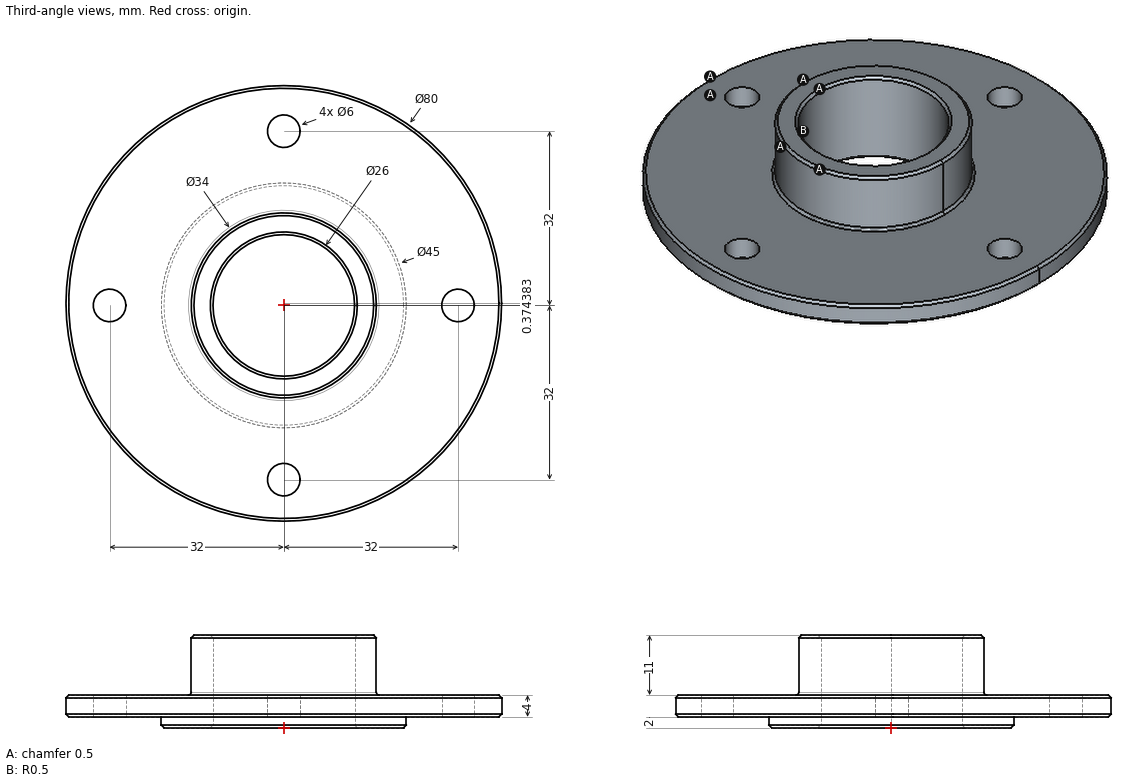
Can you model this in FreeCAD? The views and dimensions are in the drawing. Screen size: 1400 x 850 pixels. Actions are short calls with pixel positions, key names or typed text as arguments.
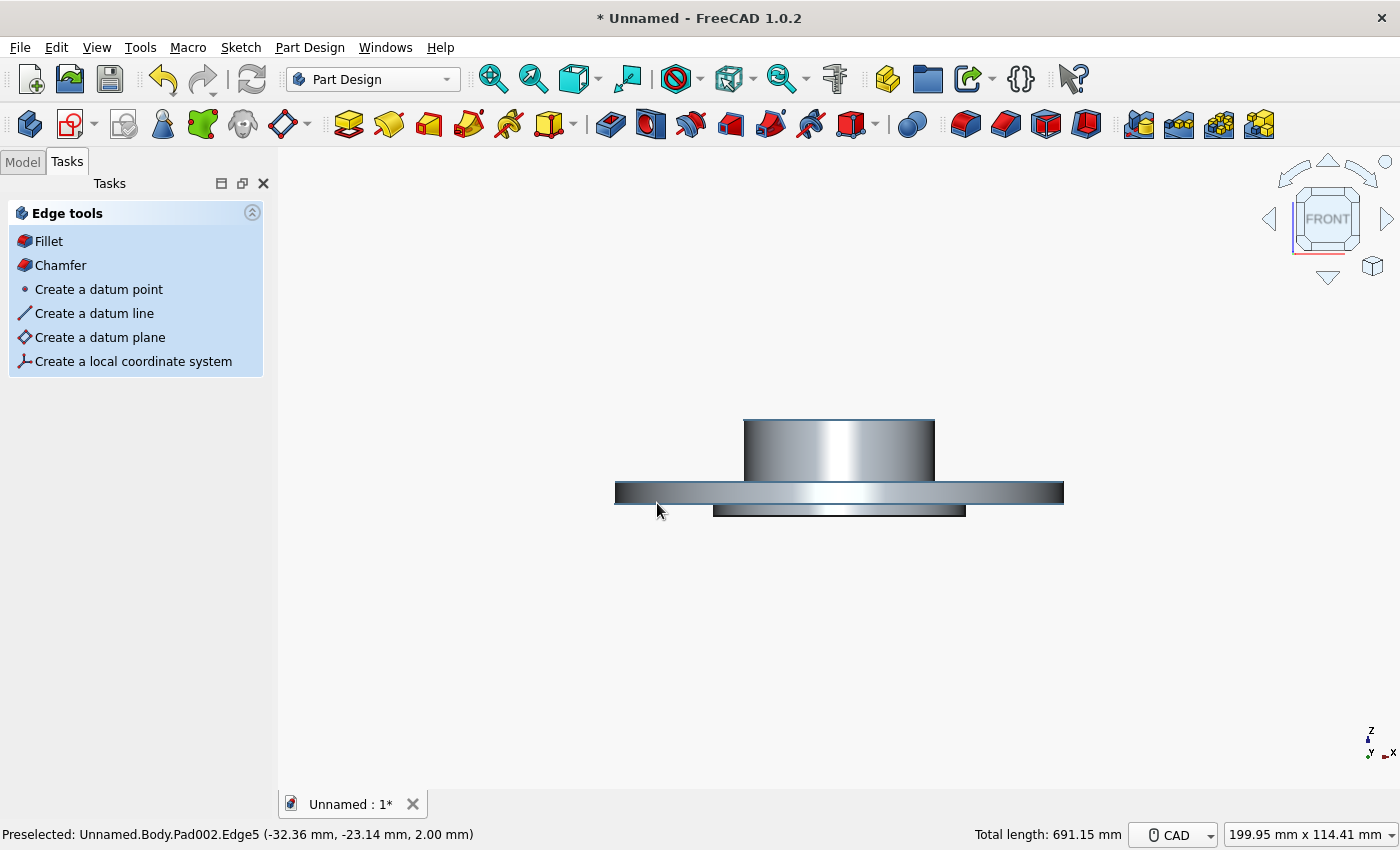
click(737, 515, ctrl)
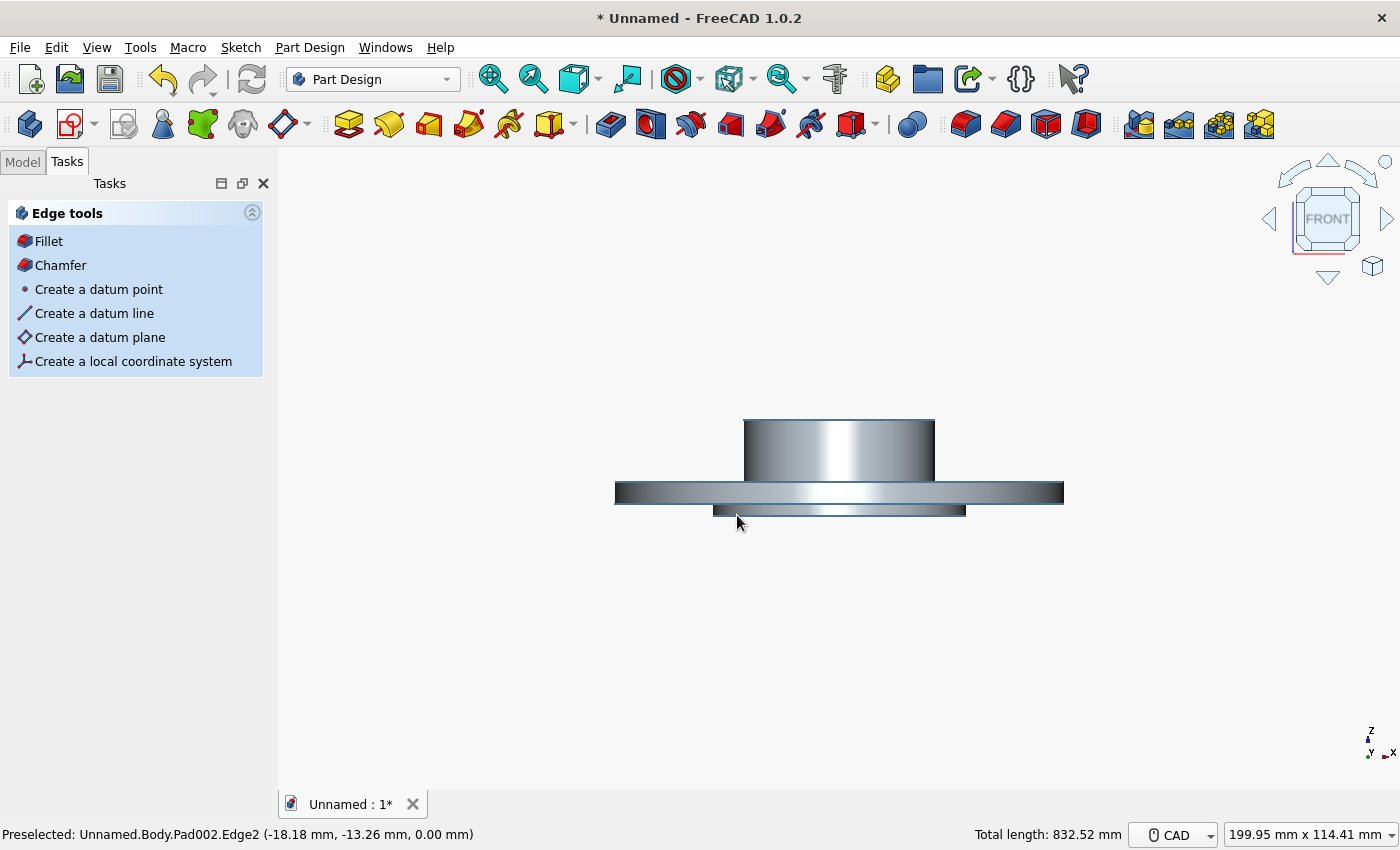
key(3)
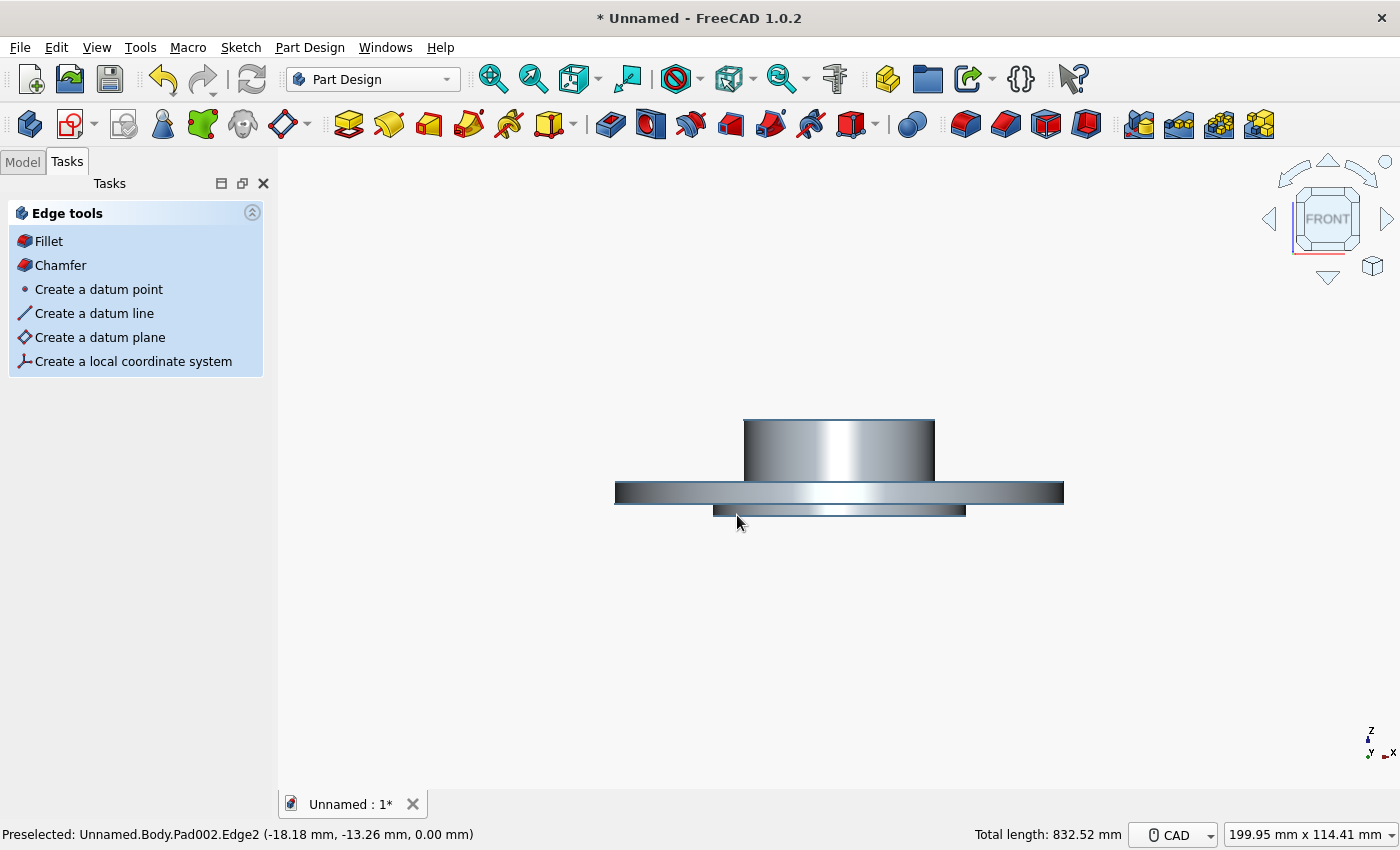
click(494, 80)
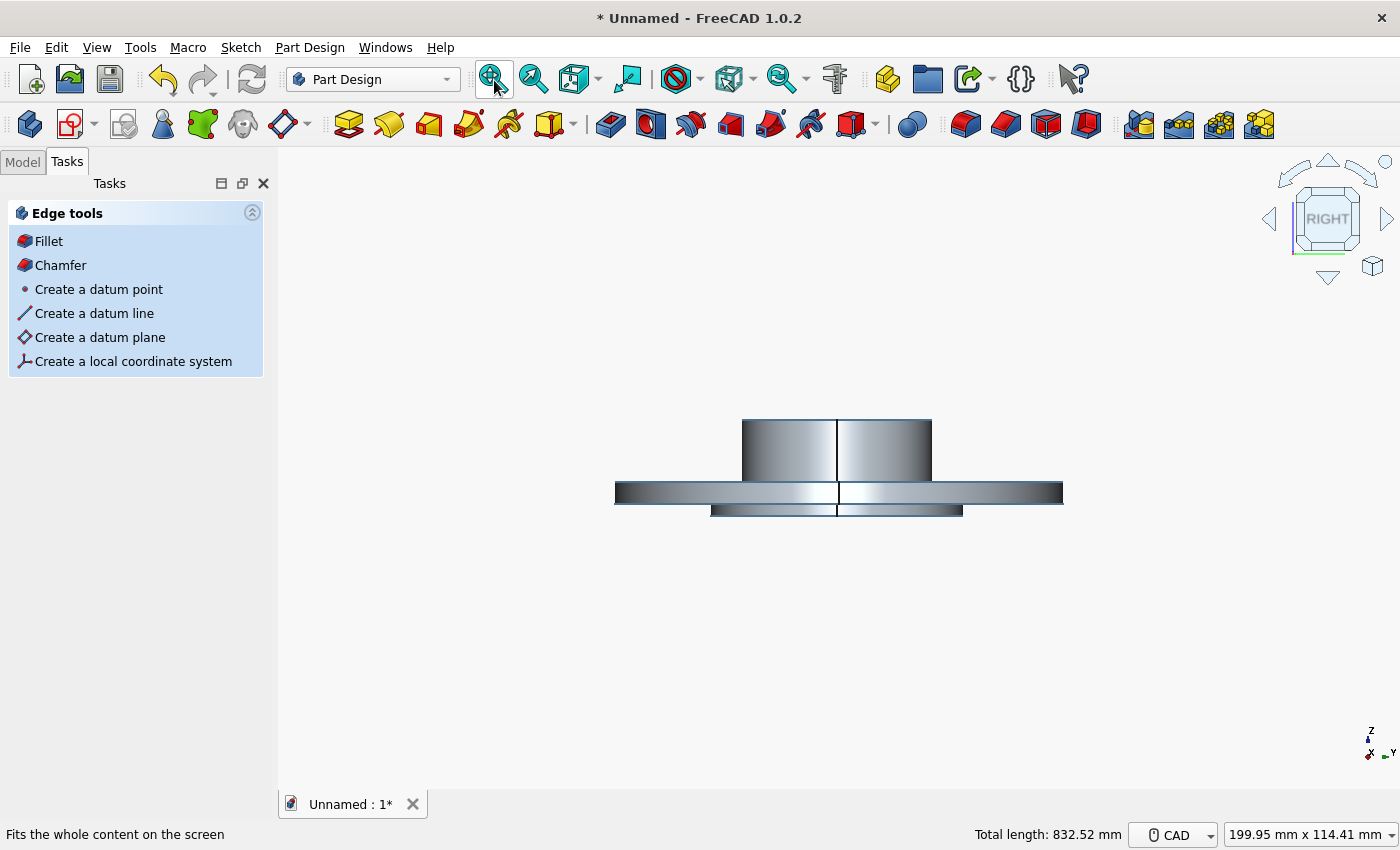
key(5)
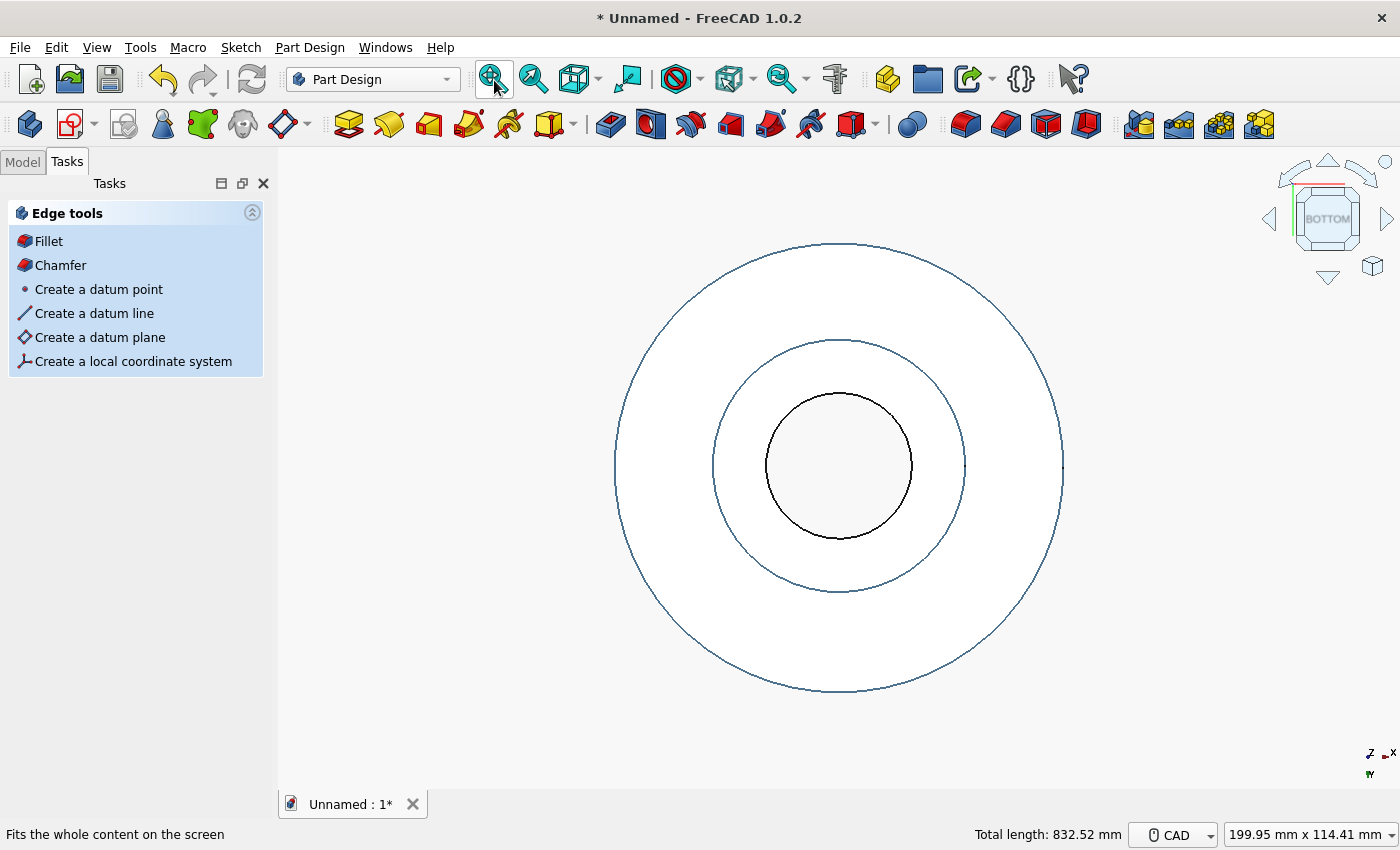
click(766, 465, ctrl)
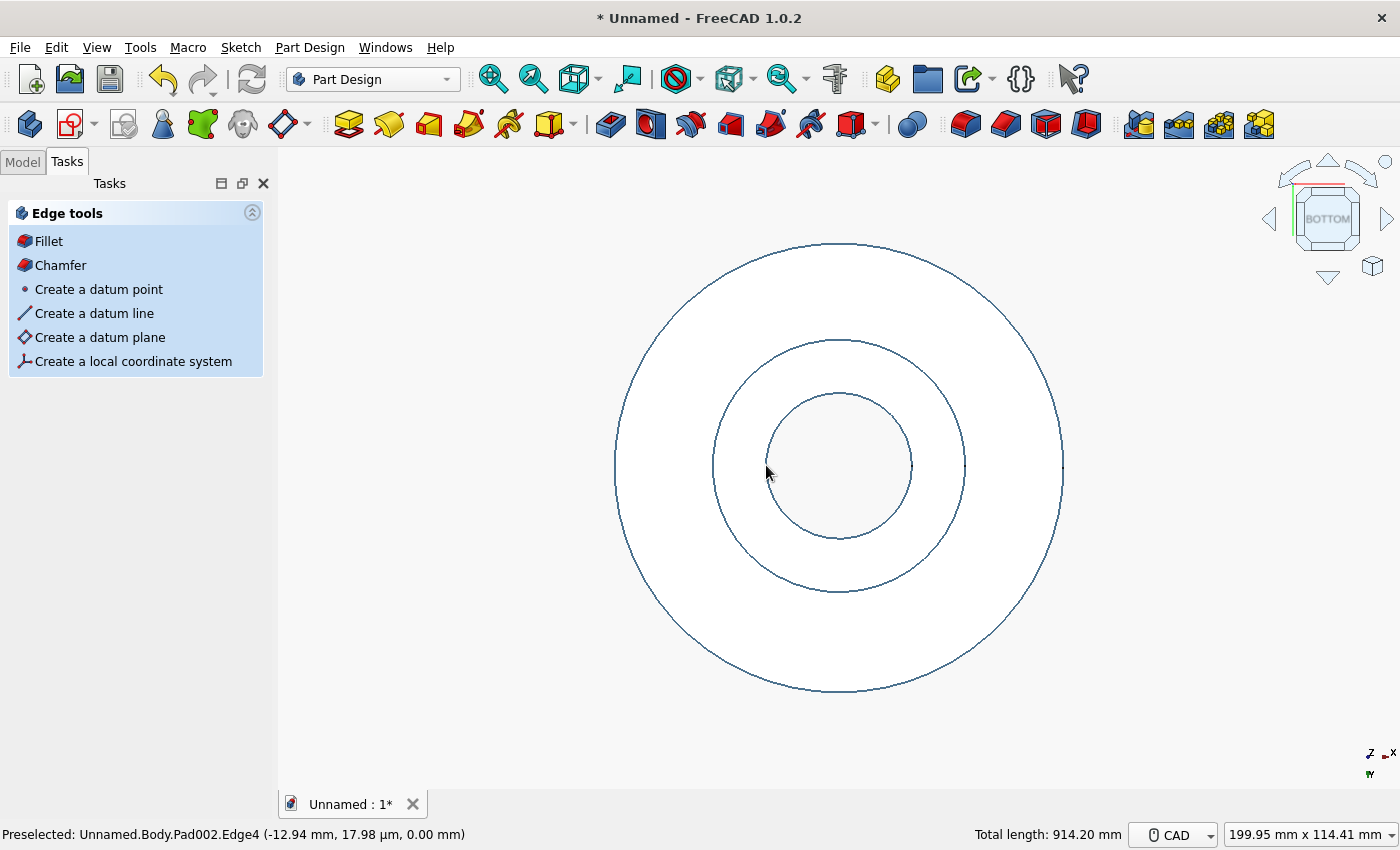
click(1006, 124)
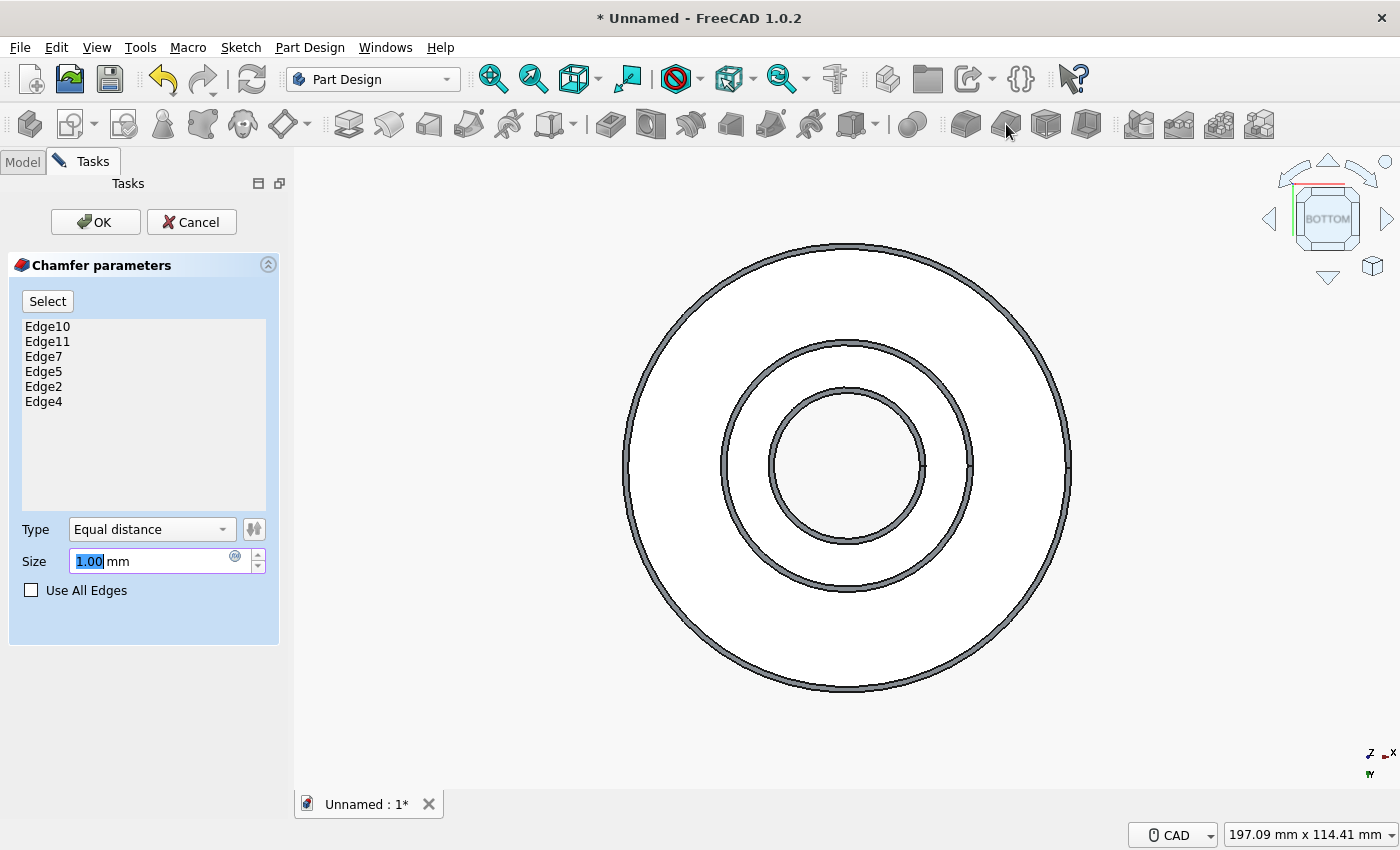
text(0.5)
key(Tab)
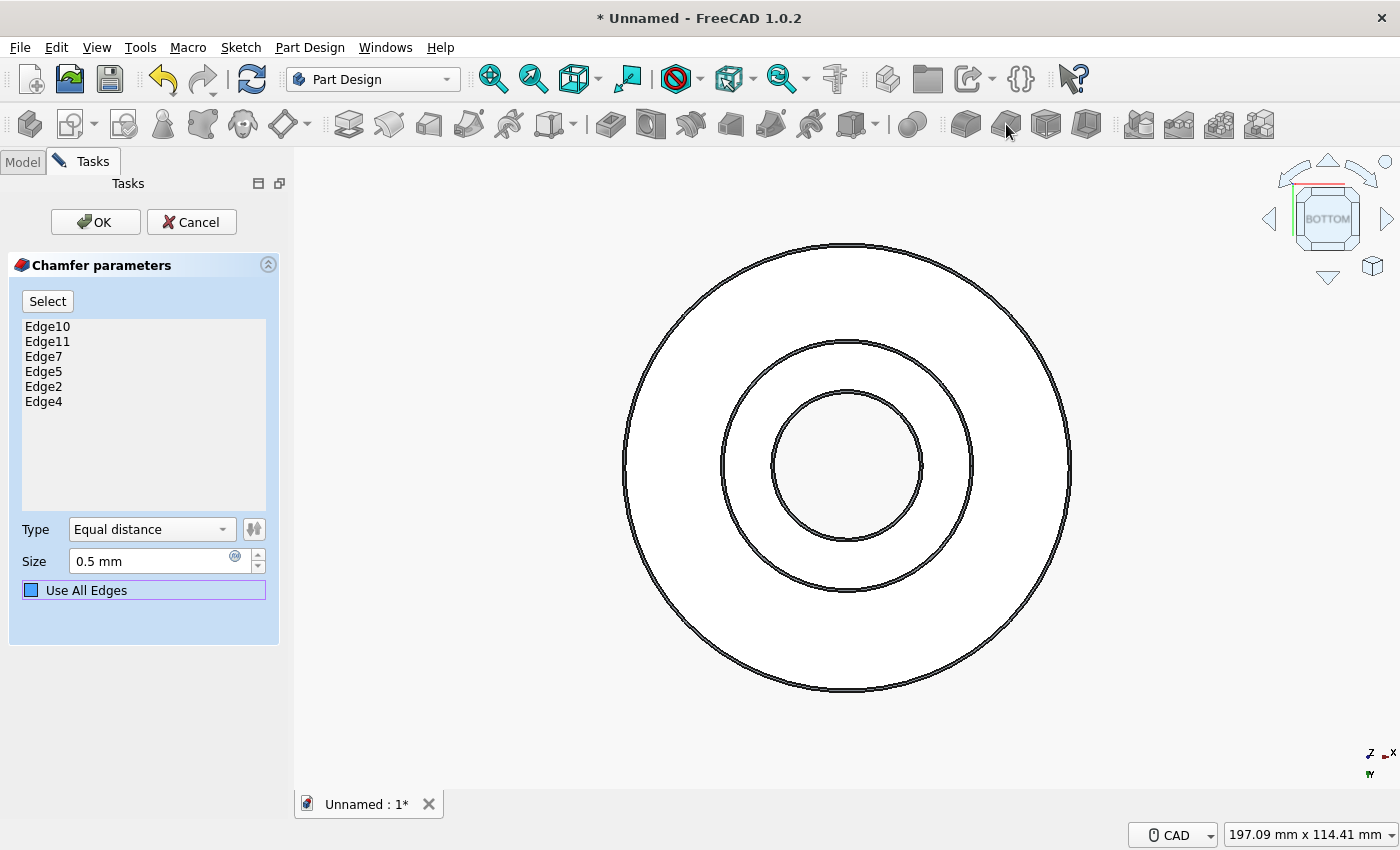
click(96, 222)